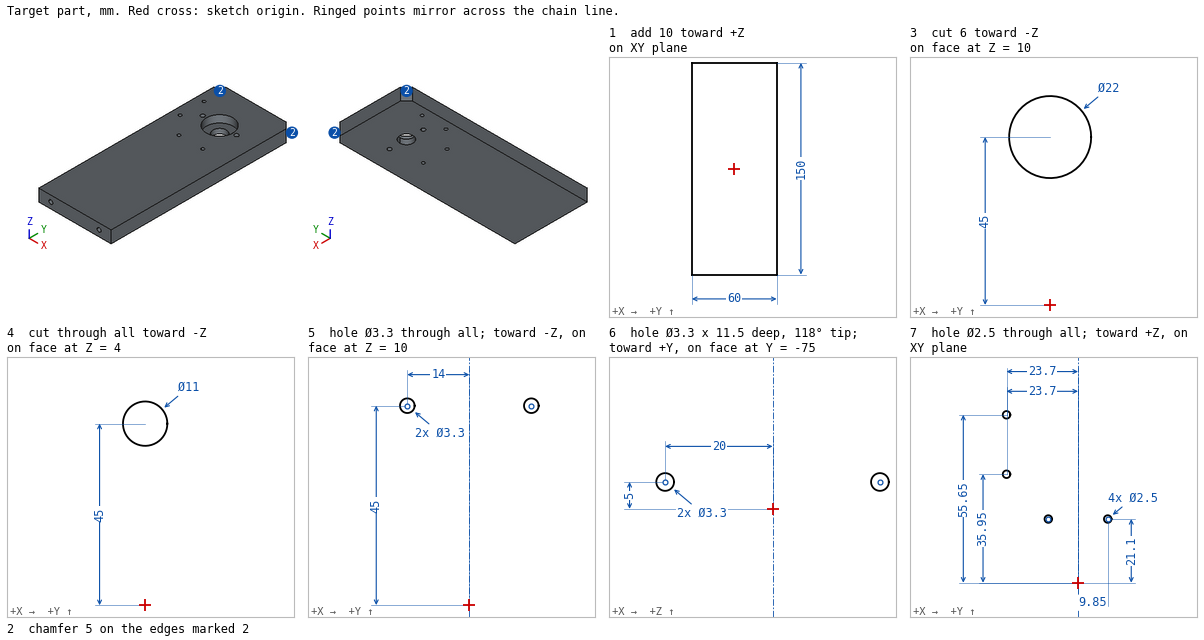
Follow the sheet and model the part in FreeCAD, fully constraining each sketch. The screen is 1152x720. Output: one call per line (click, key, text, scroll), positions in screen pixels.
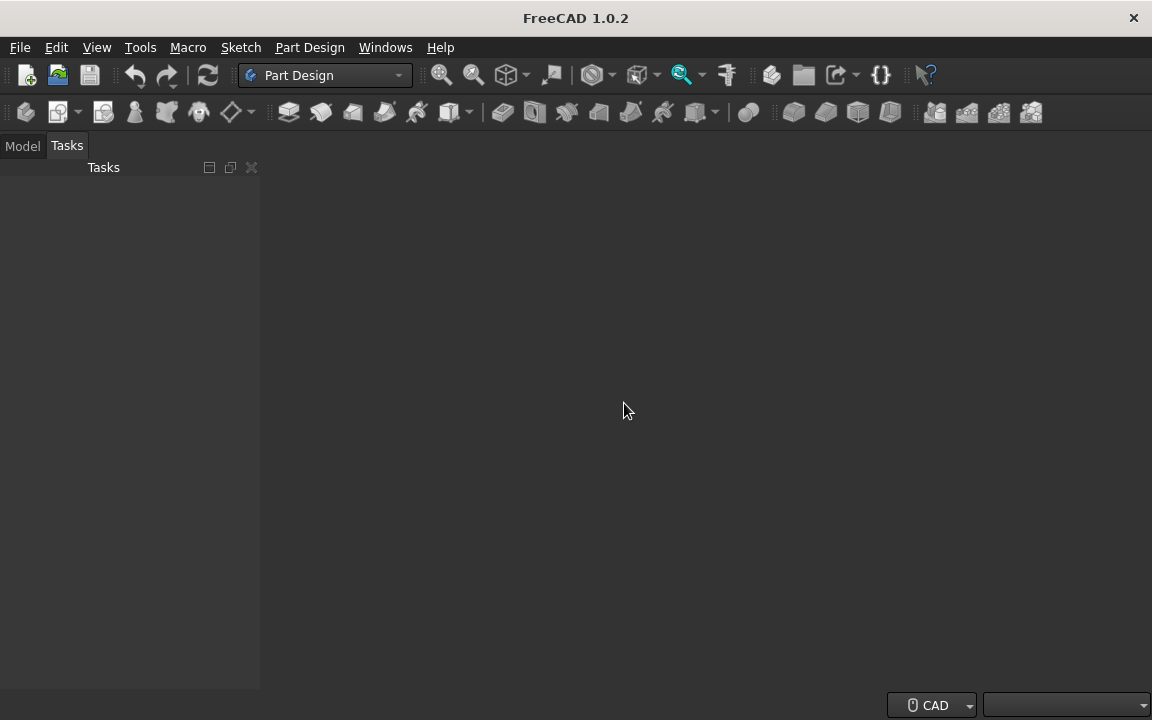
click(26, 76)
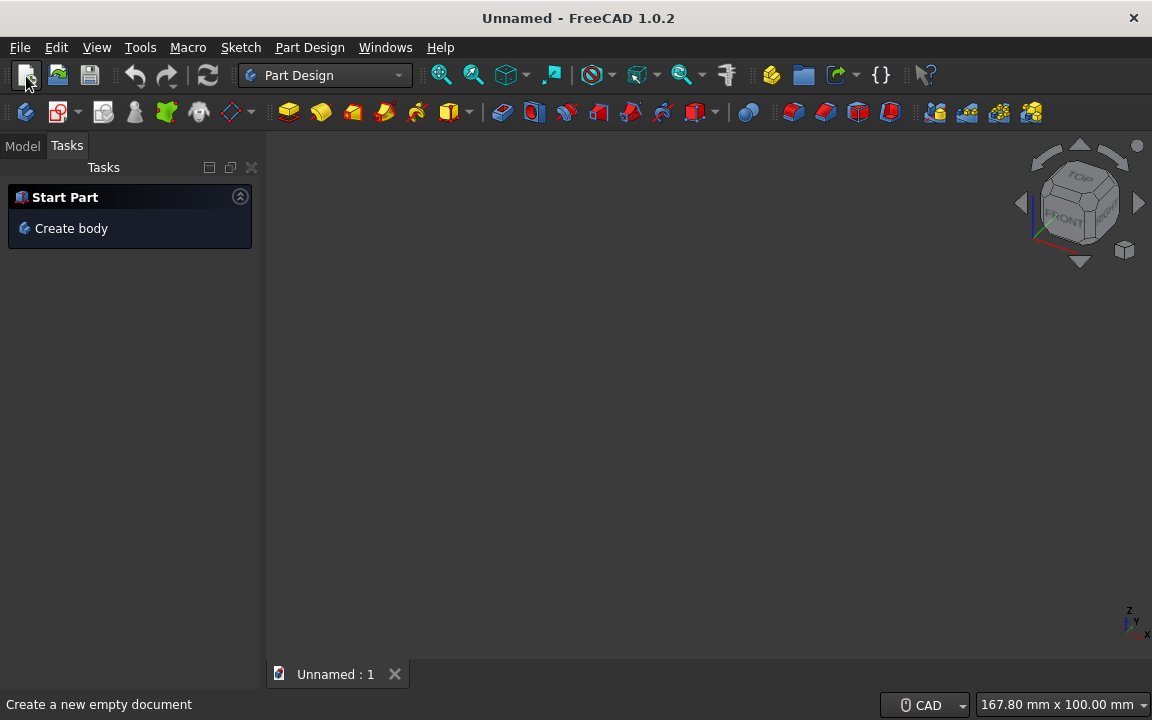
click(58, 112)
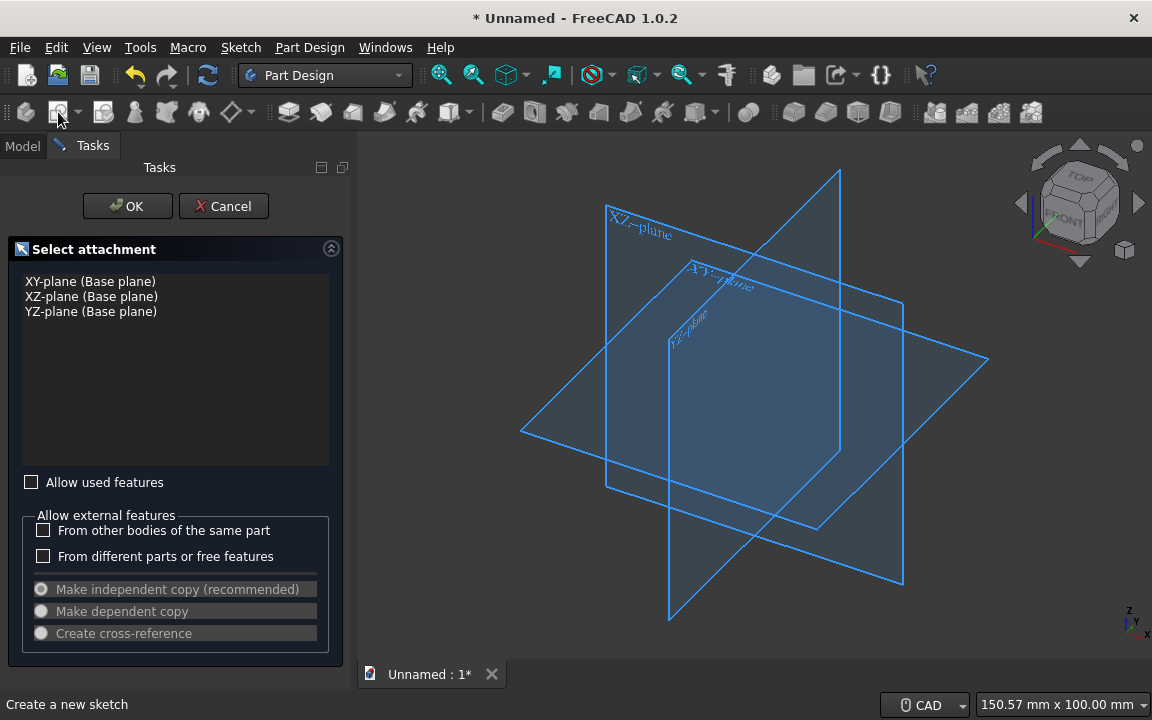
click(82, 282)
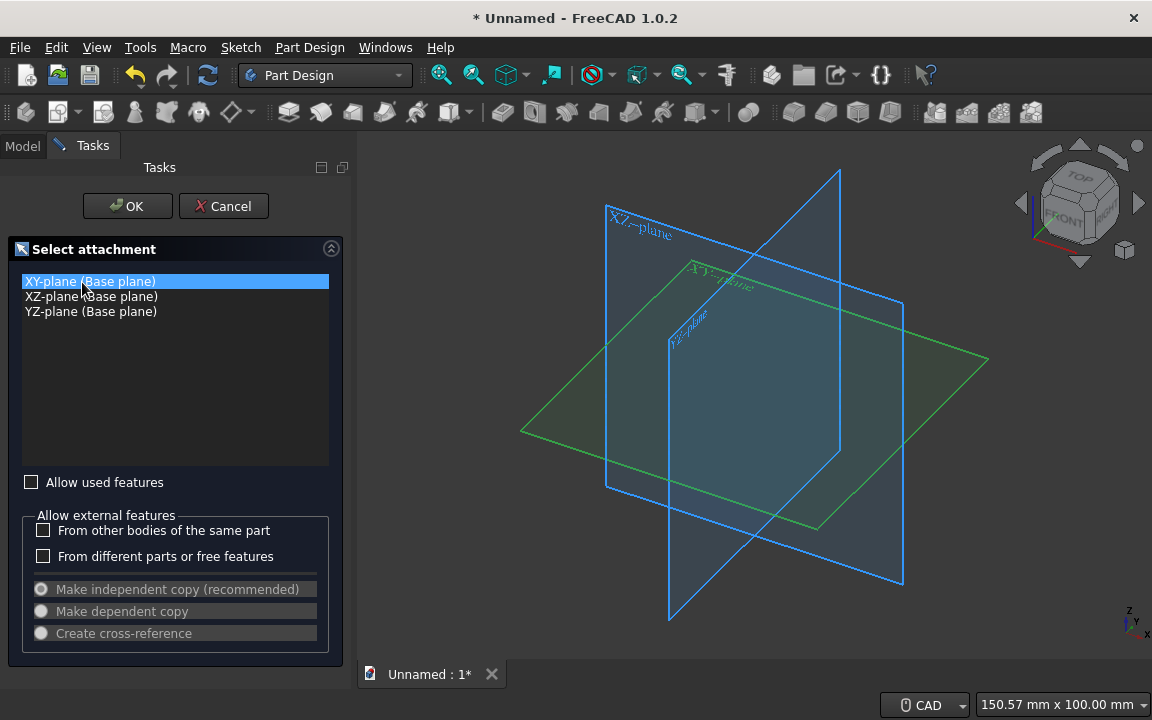
click(128, 206)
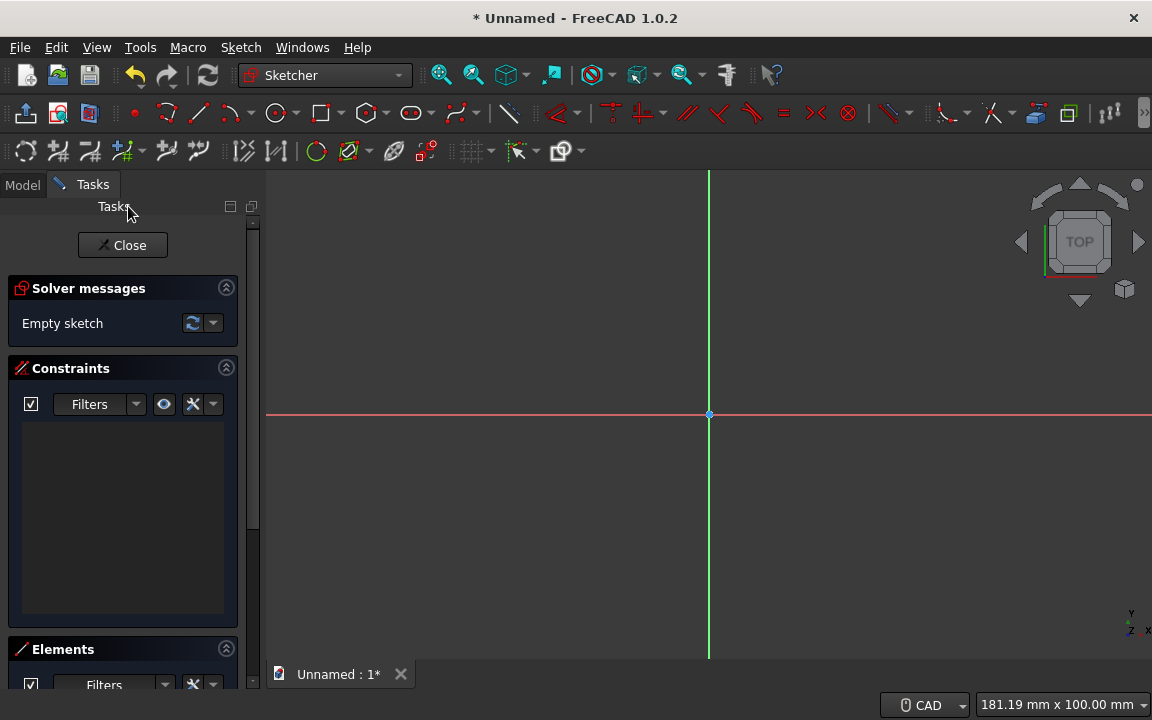
scroll(585, 414, down, 4)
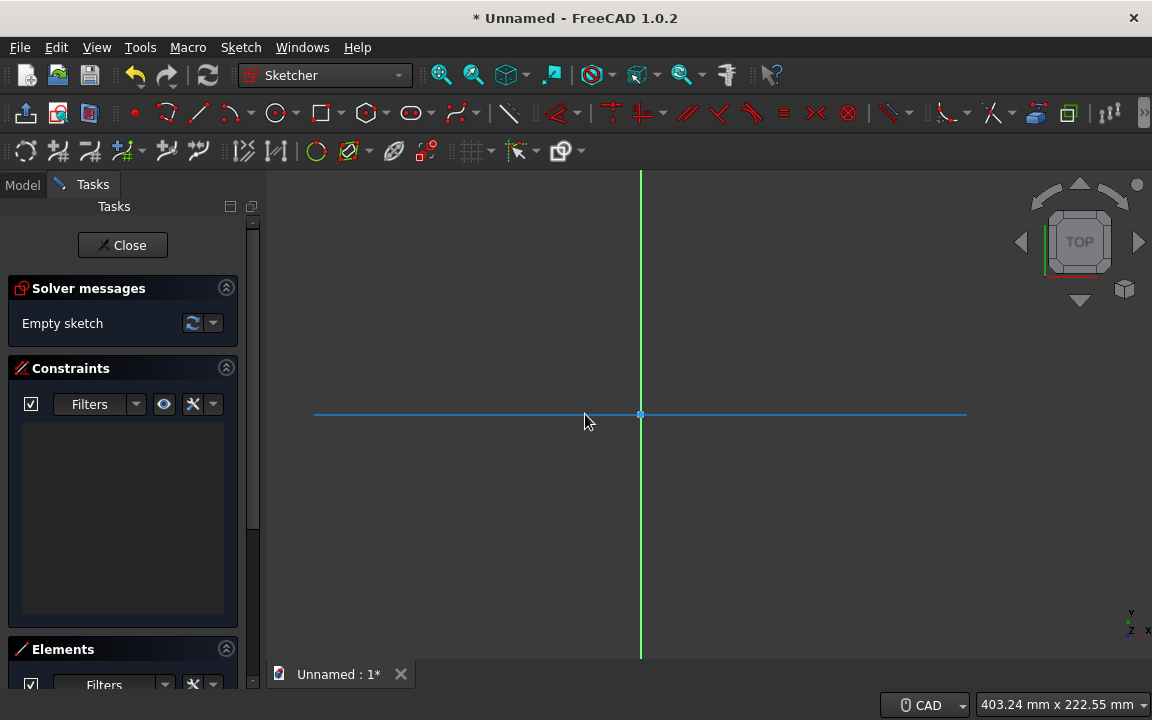
key(g)
key(v)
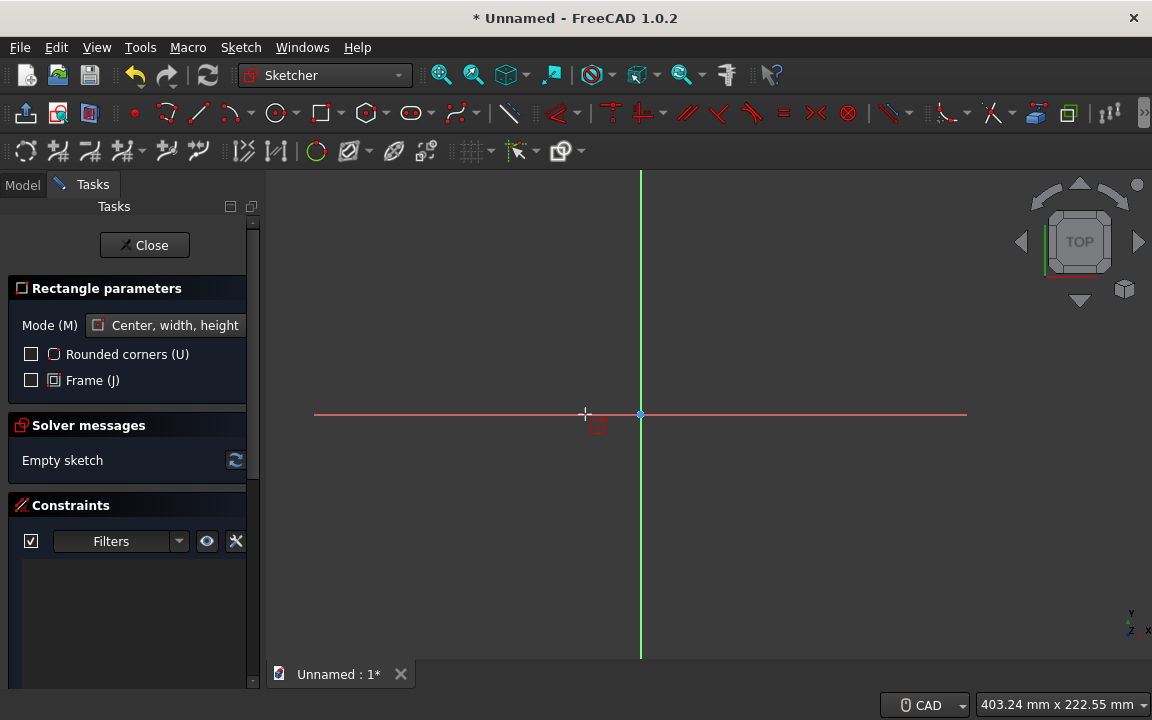
click(641, 414)
click(707, 250)
key(Escape)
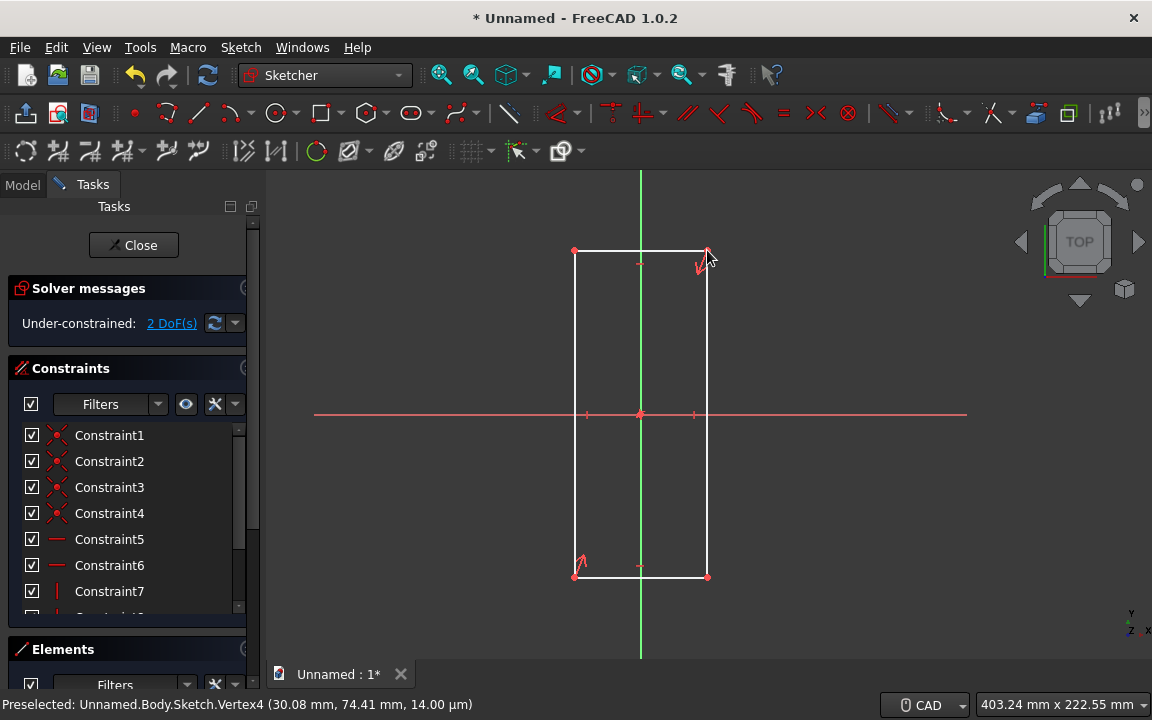
click(556, 114)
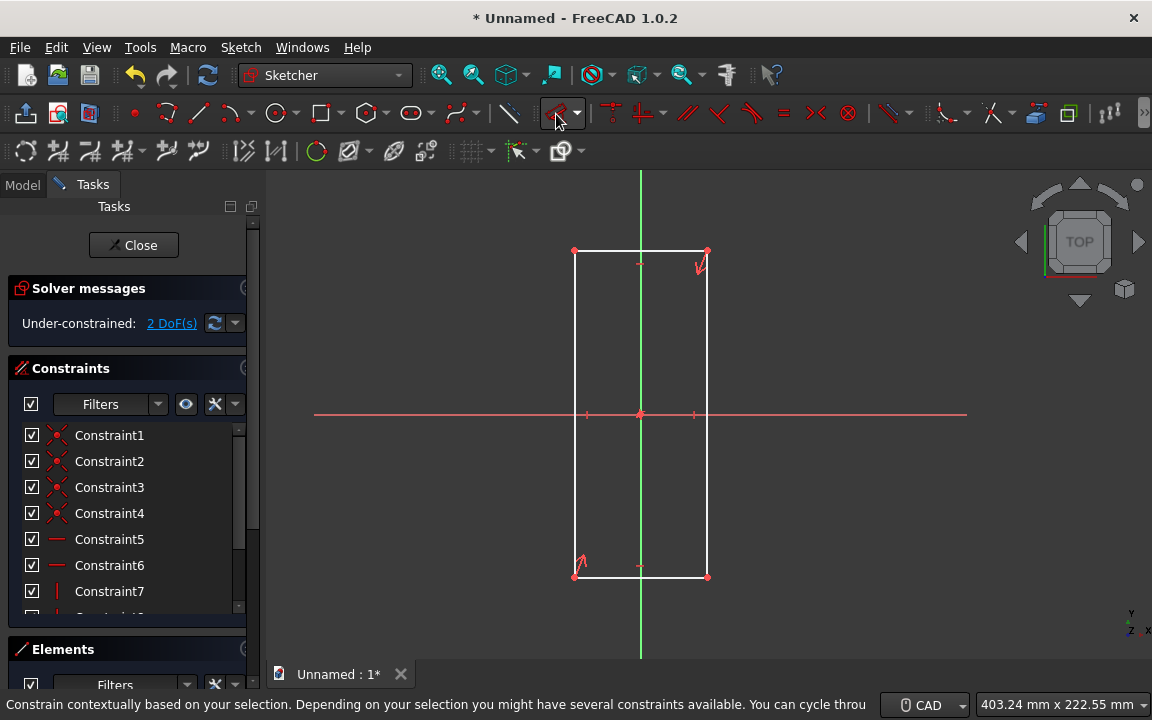
click(614, 578)
click(611, 612)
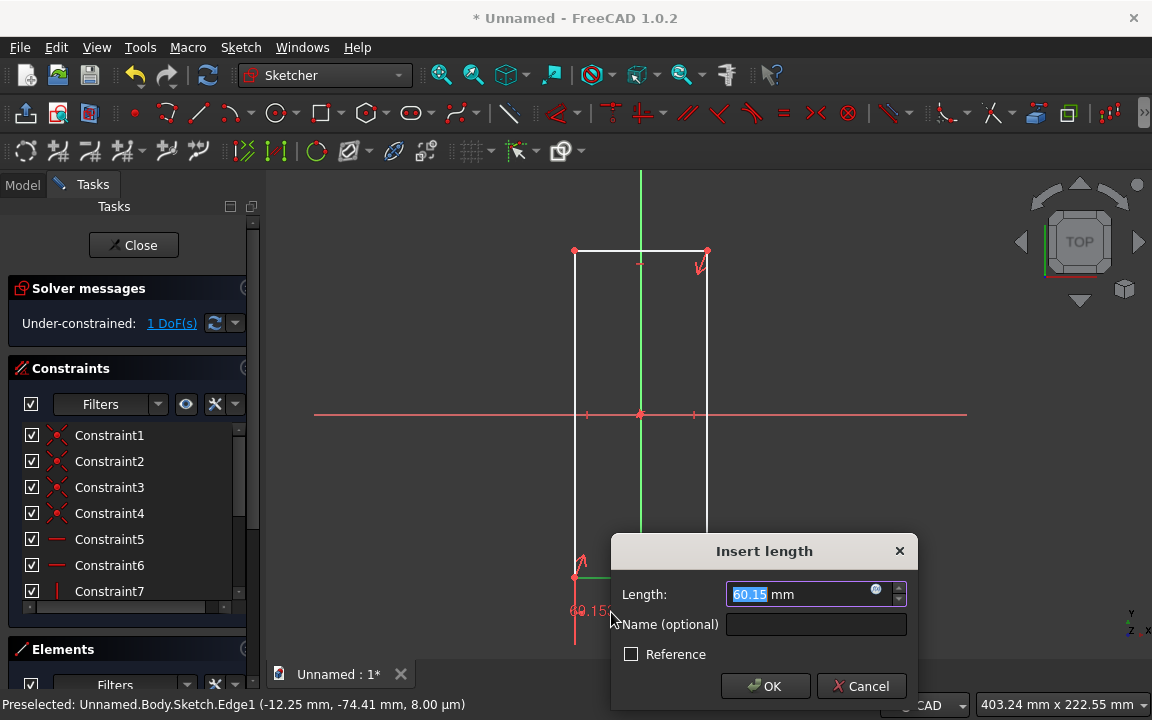
text(60)
key(Return)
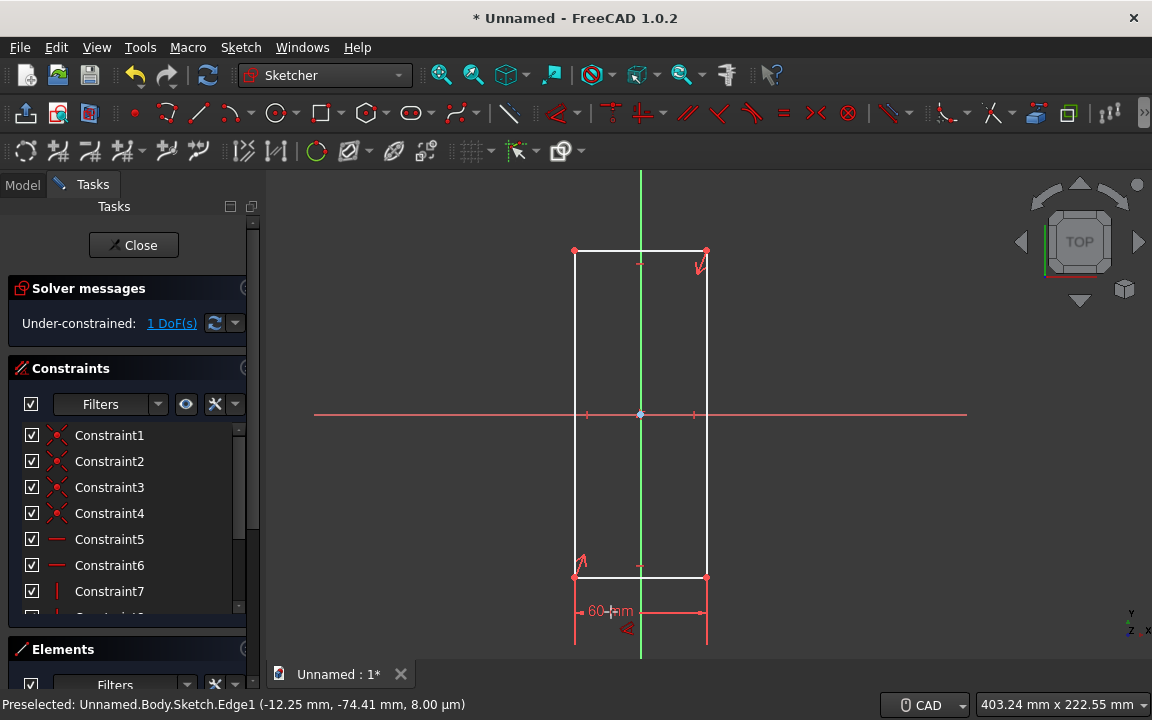
click(707, 480)
click(741, 339)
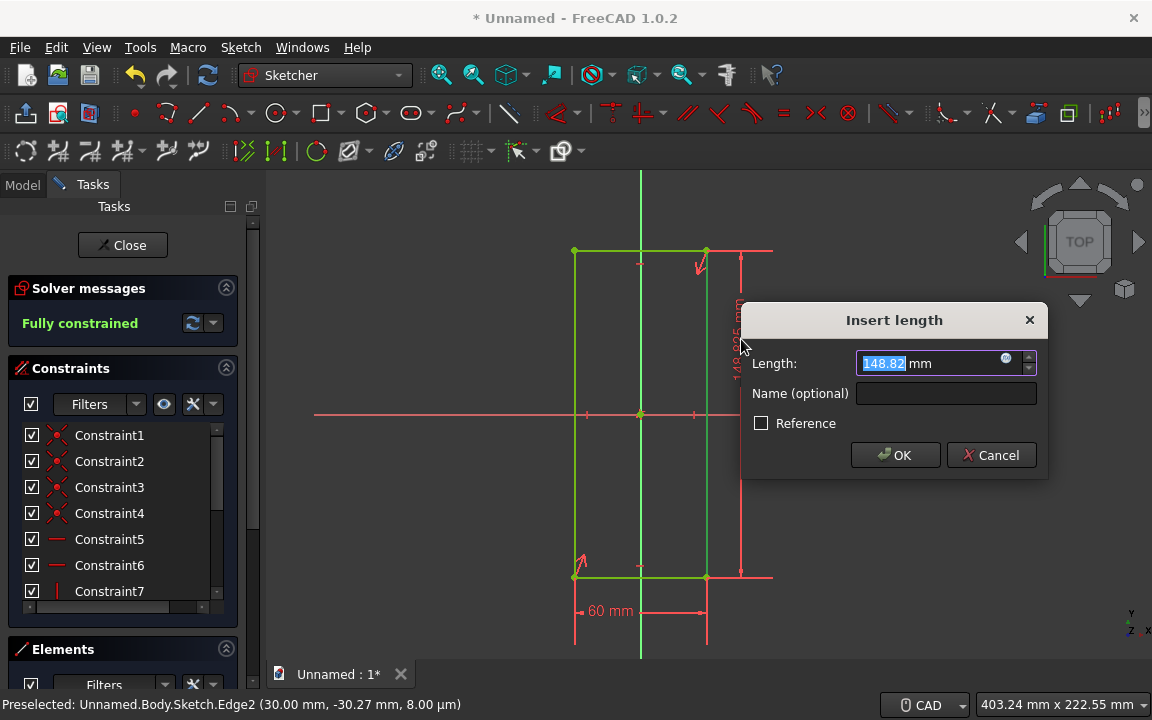
text(150)
key(Return)
key(Escape)